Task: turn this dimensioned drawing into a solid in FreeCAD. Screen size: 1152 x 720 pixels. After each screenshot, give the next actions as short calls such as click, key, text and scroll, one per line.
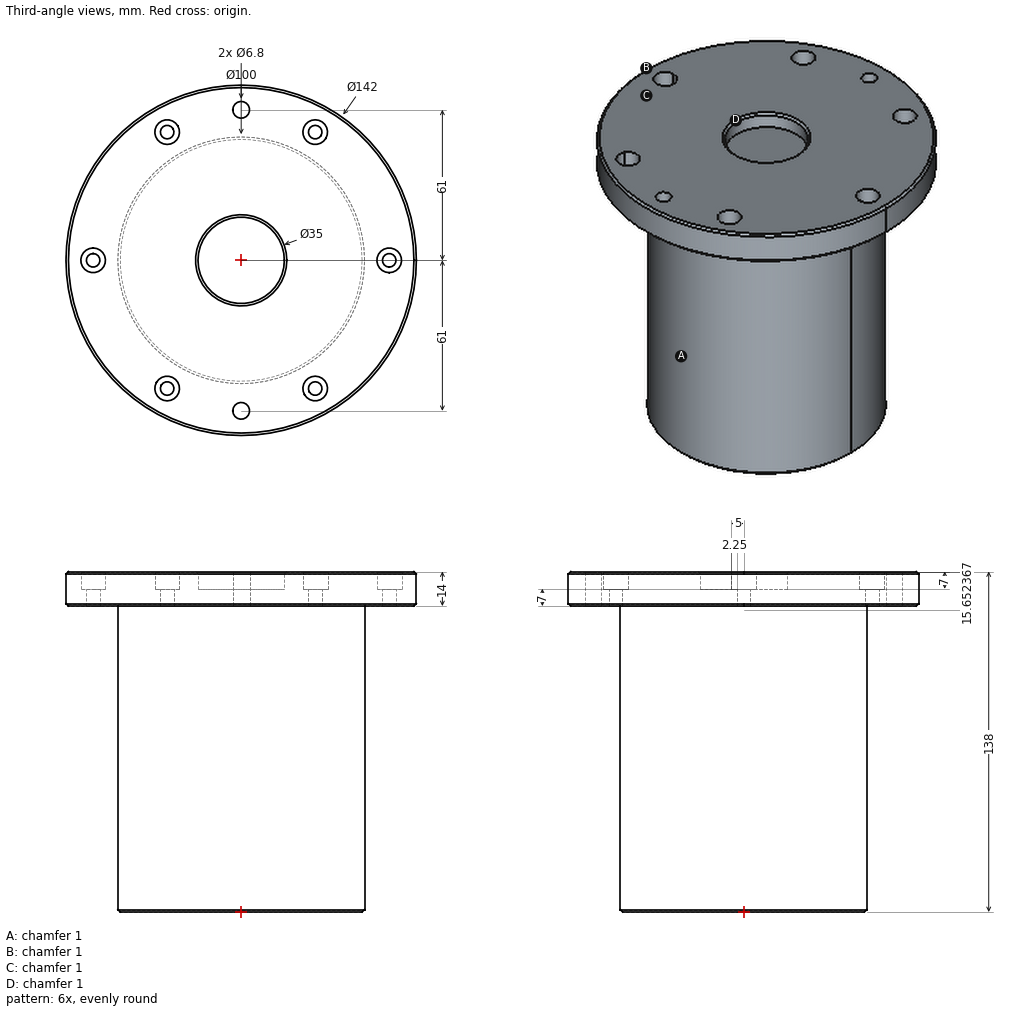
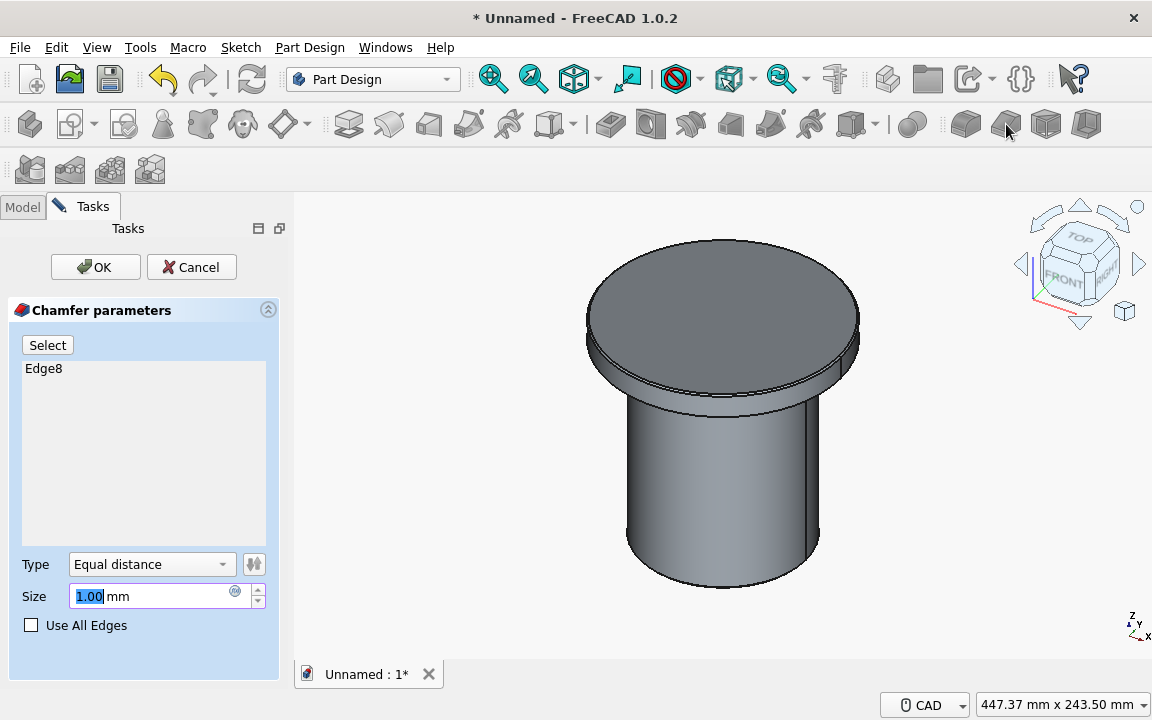
text(1)
key(Tab)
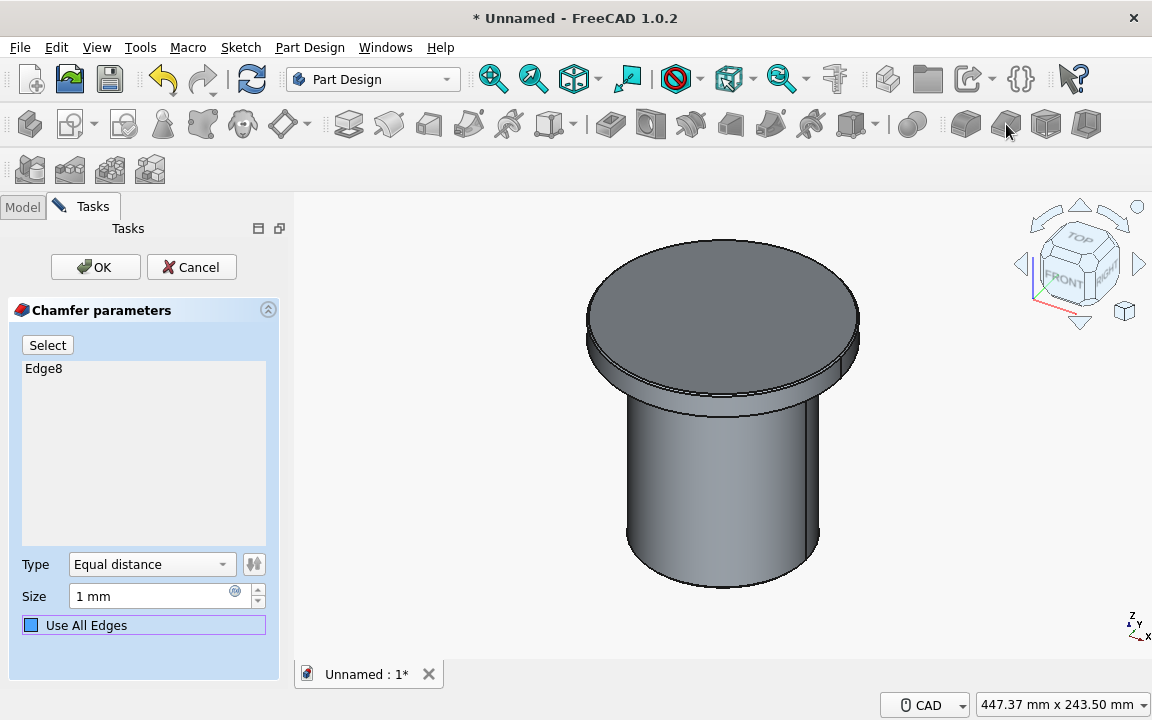
click(96, 267)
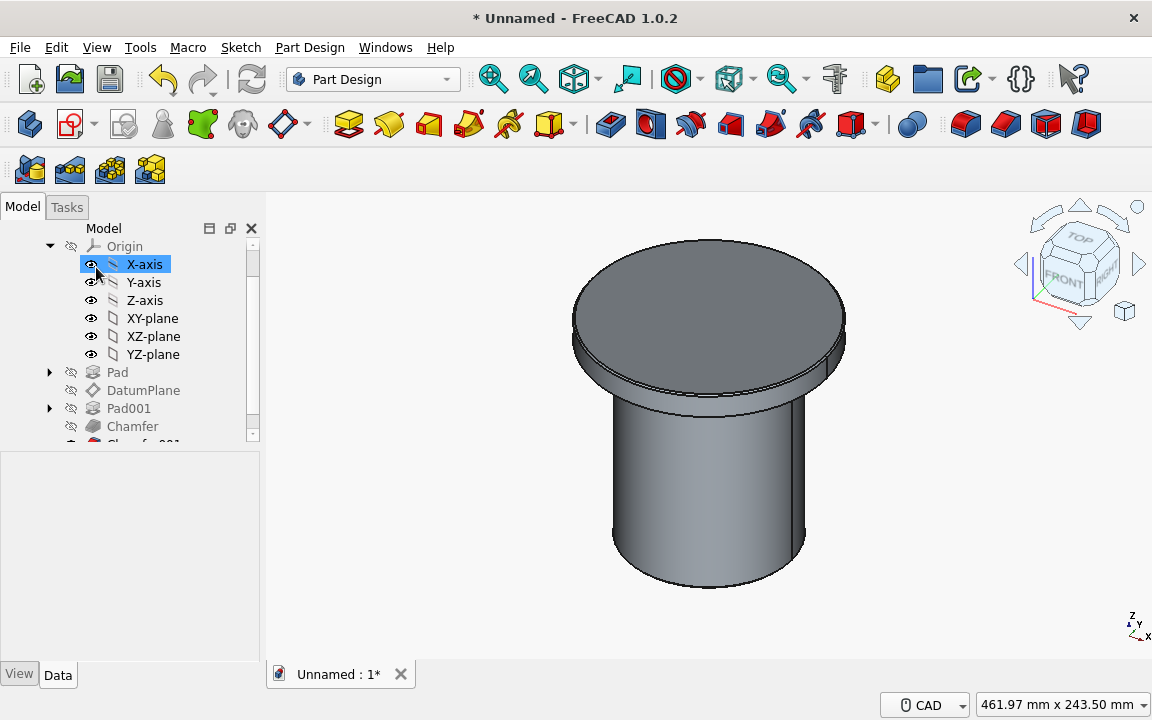
key(0)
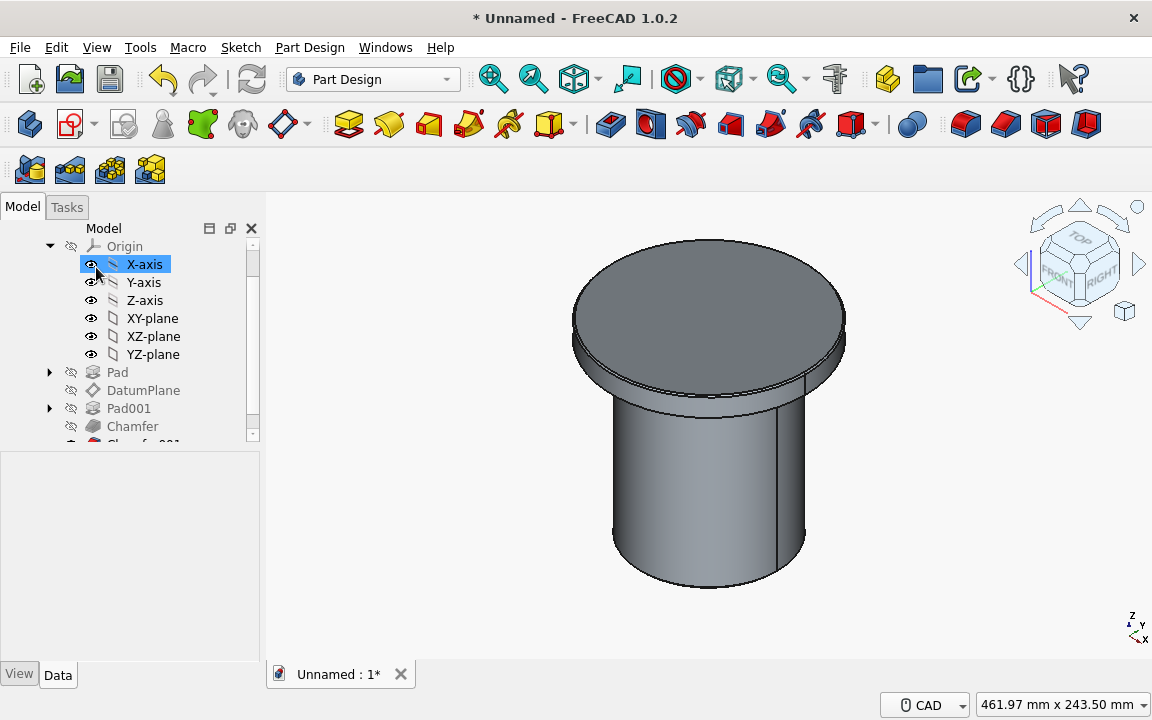
key(2)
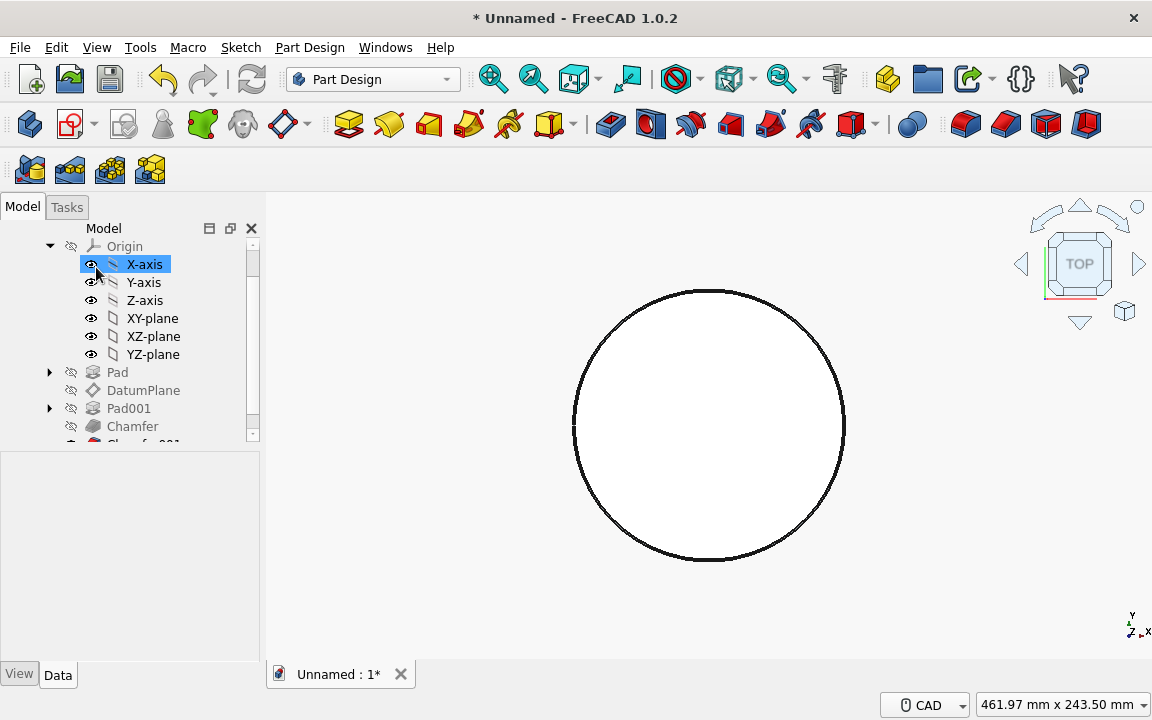
key(1)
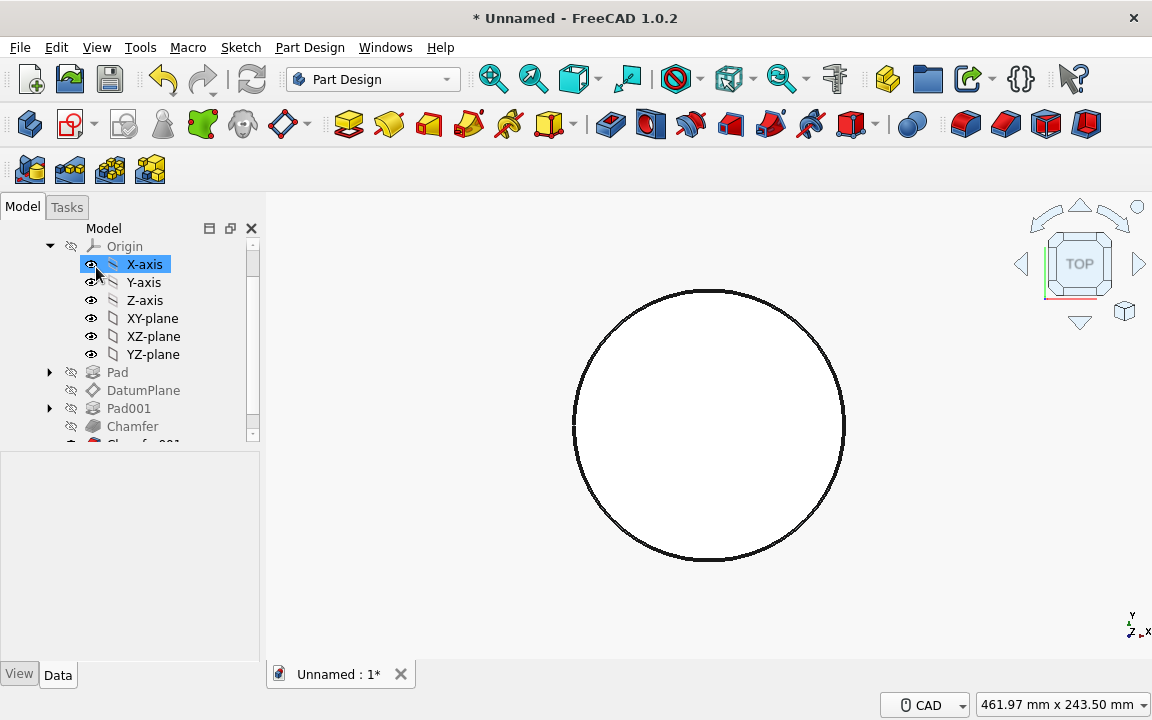
click(599, 319)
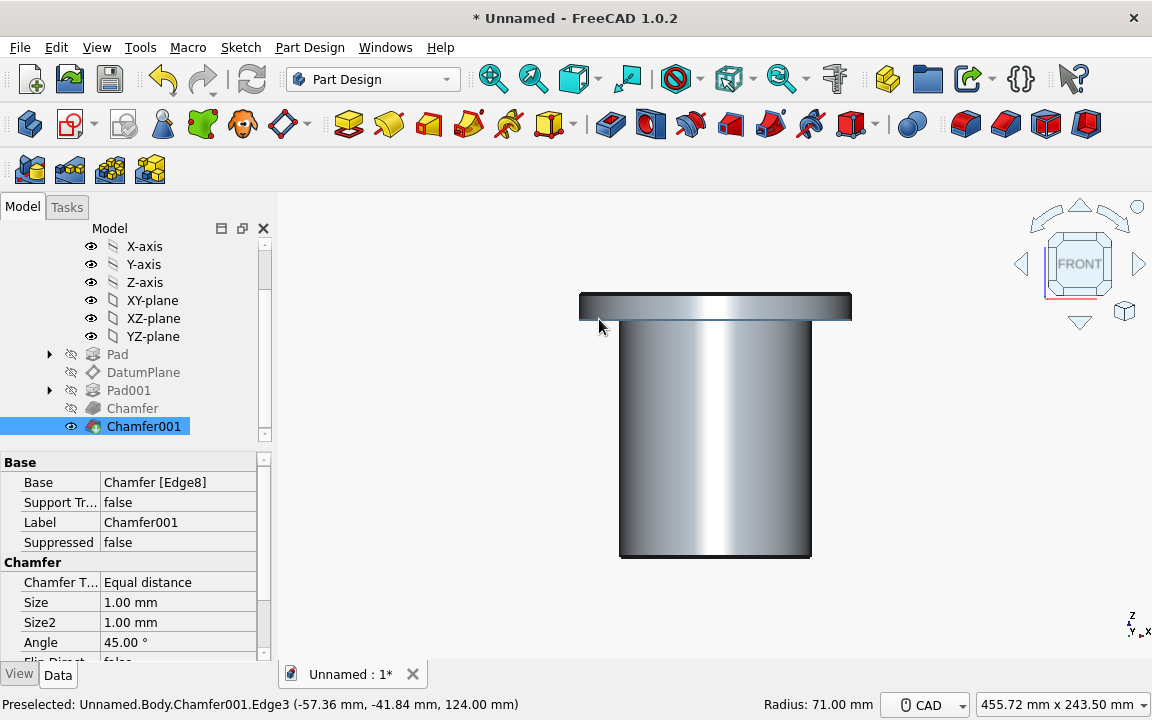
click(1006, 124)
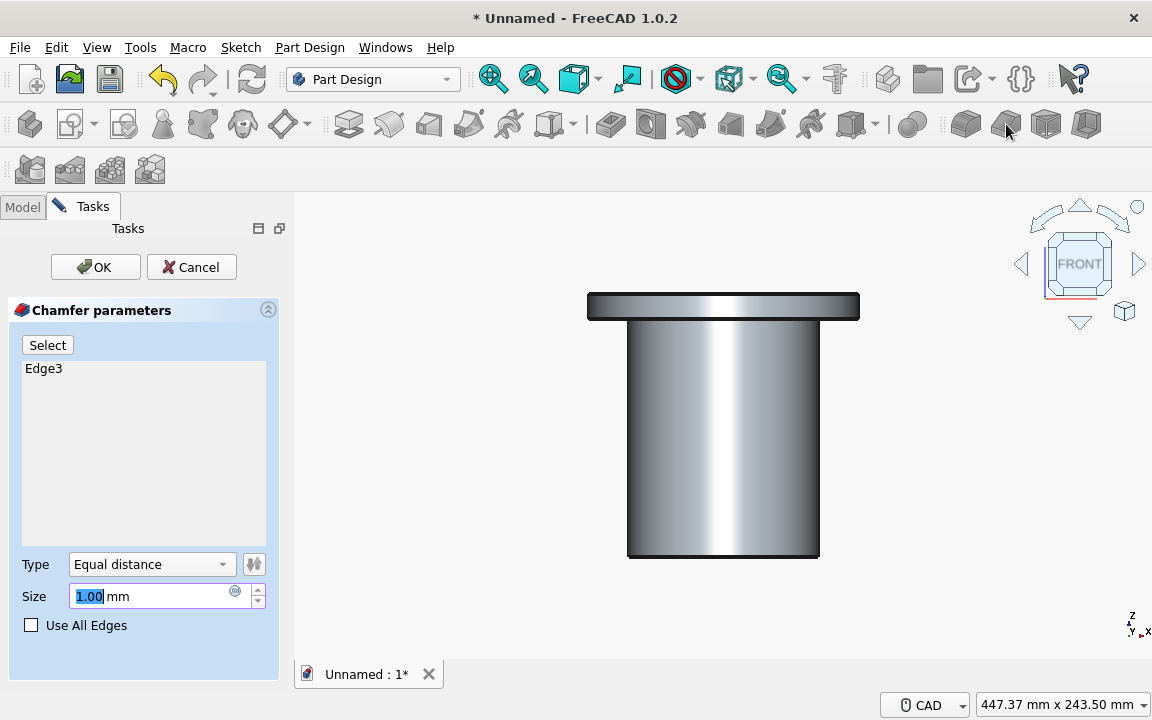
text(1)
key(Tab)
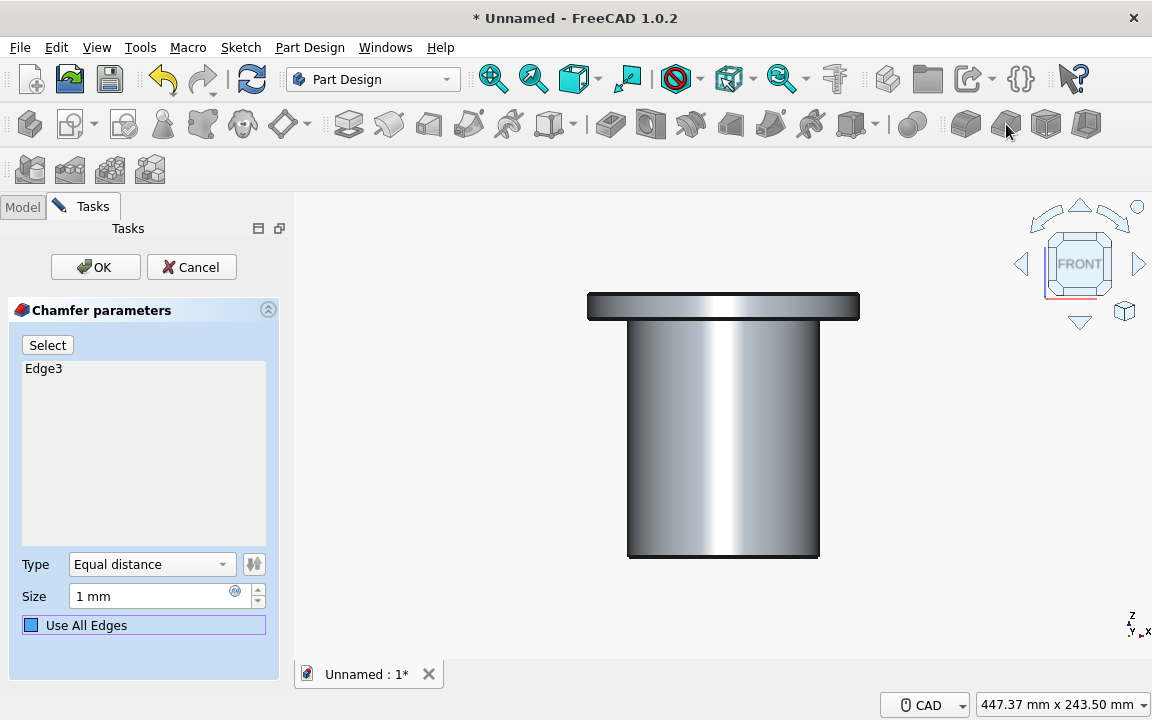
click(96, 267)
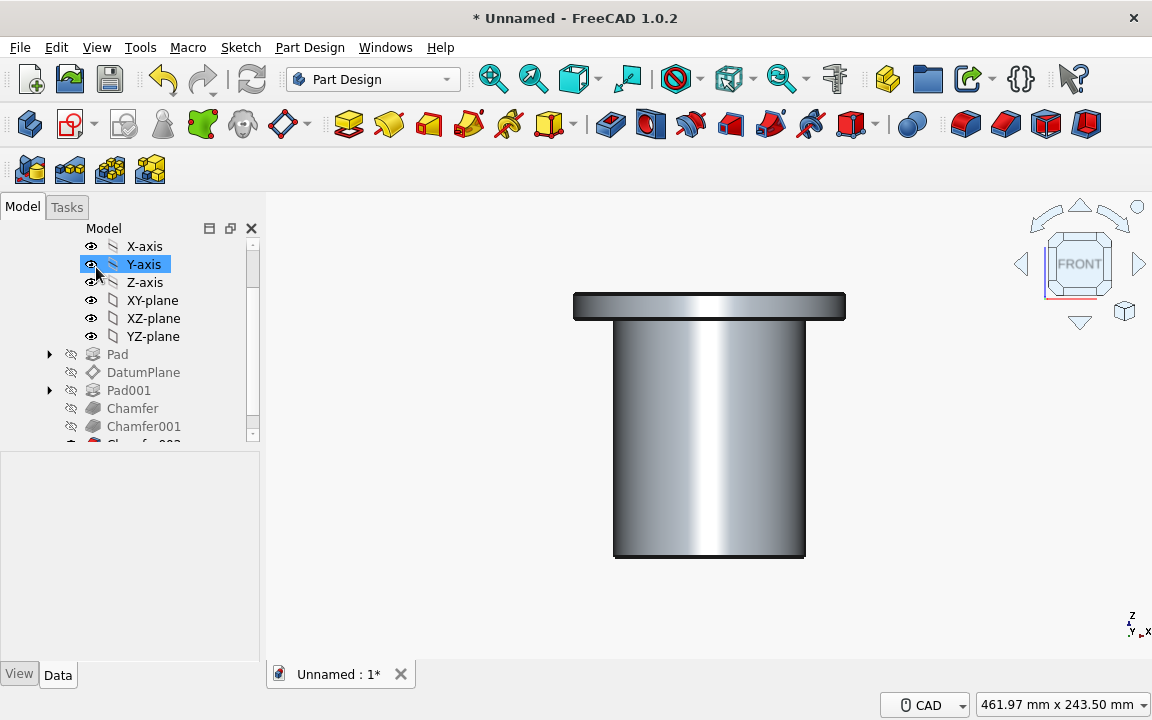
key(0)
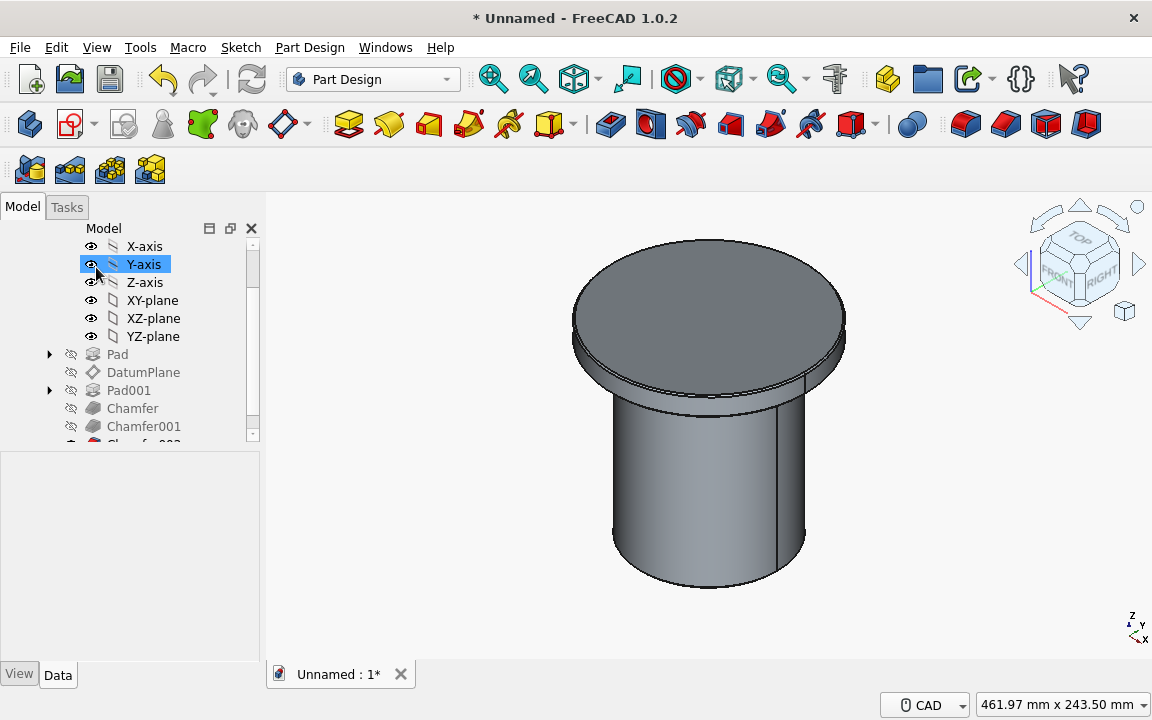
click(709, 316)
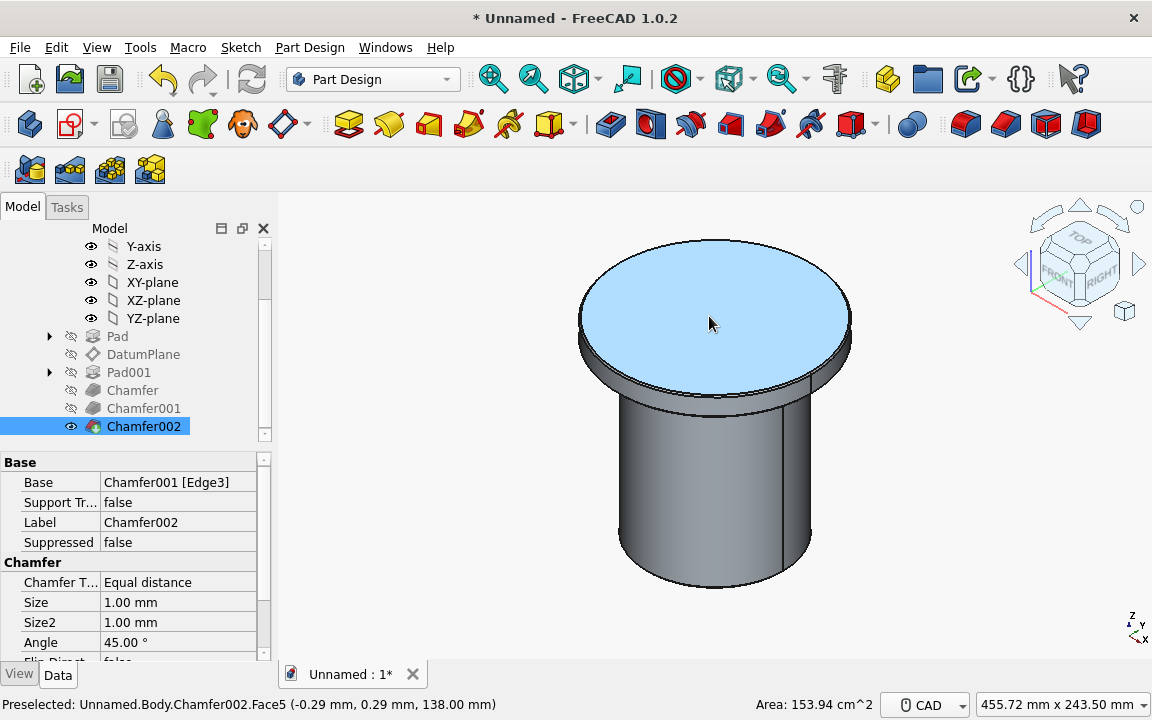
click(70, 124)